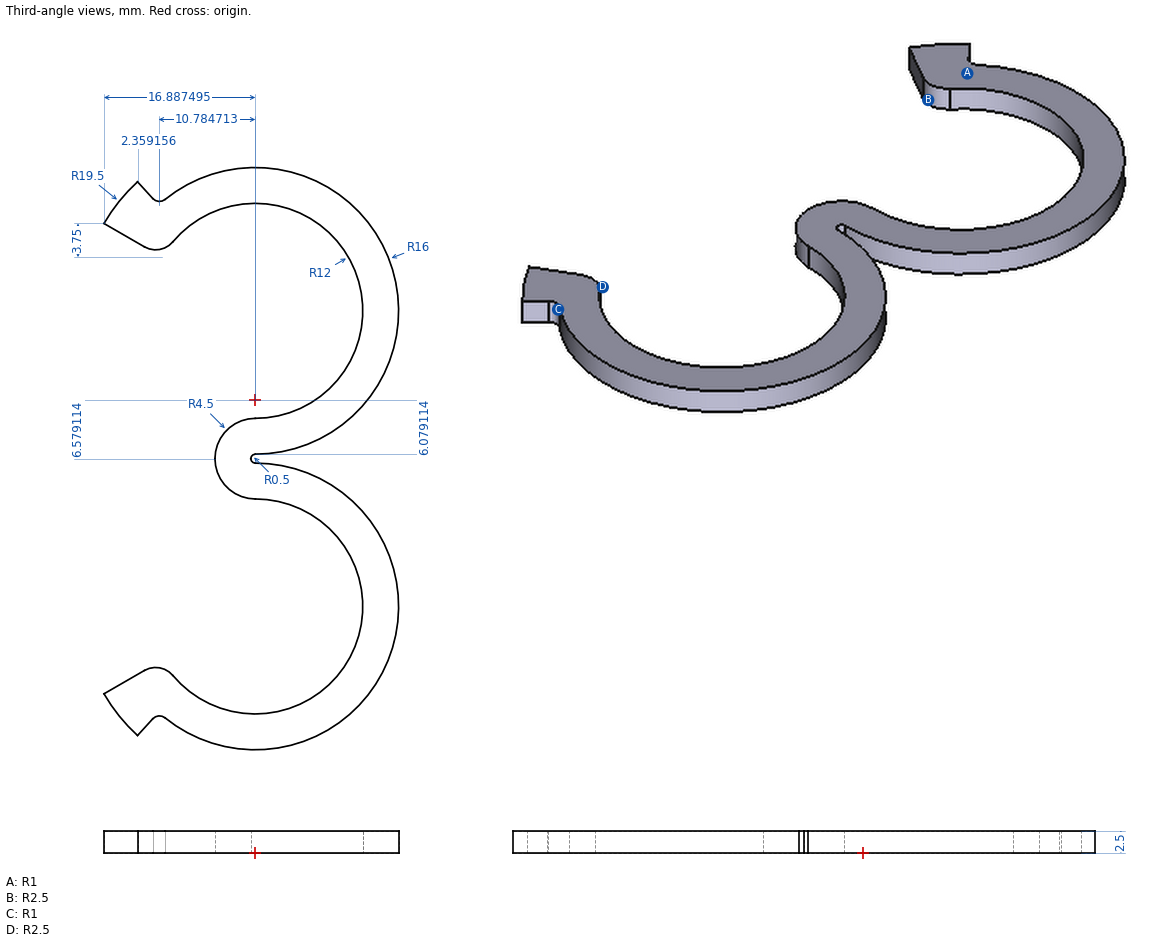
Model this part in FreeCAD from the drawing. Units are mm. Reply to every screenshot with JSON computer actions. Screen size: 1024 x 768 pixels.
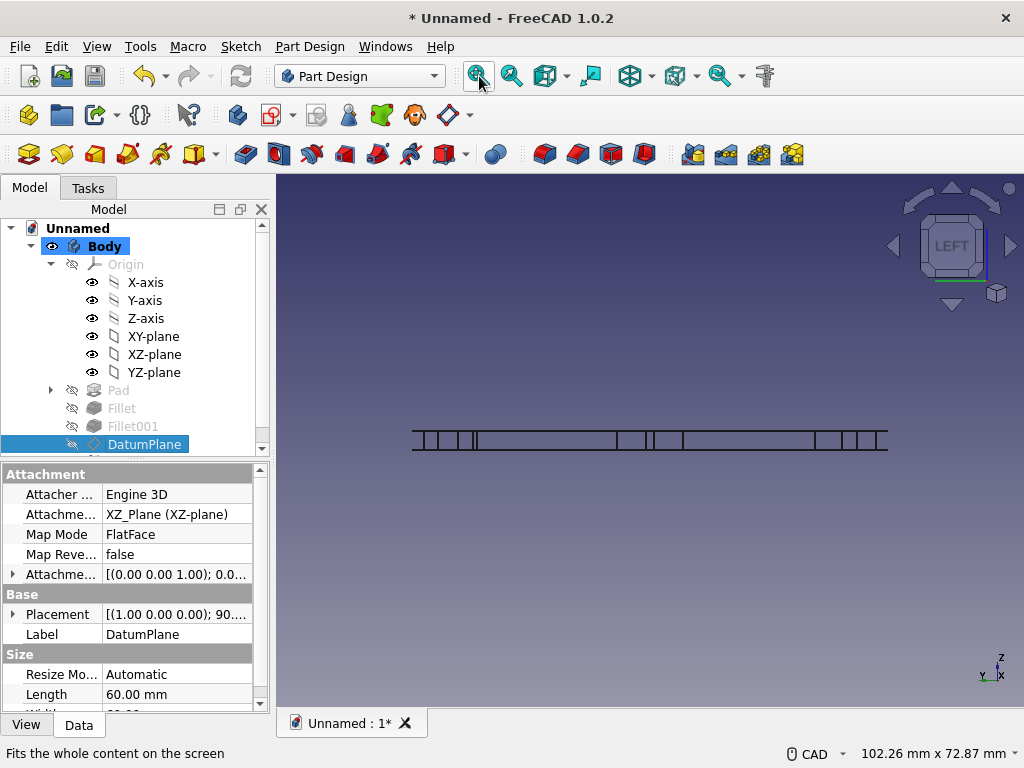
{"action": "key", "text": "0"}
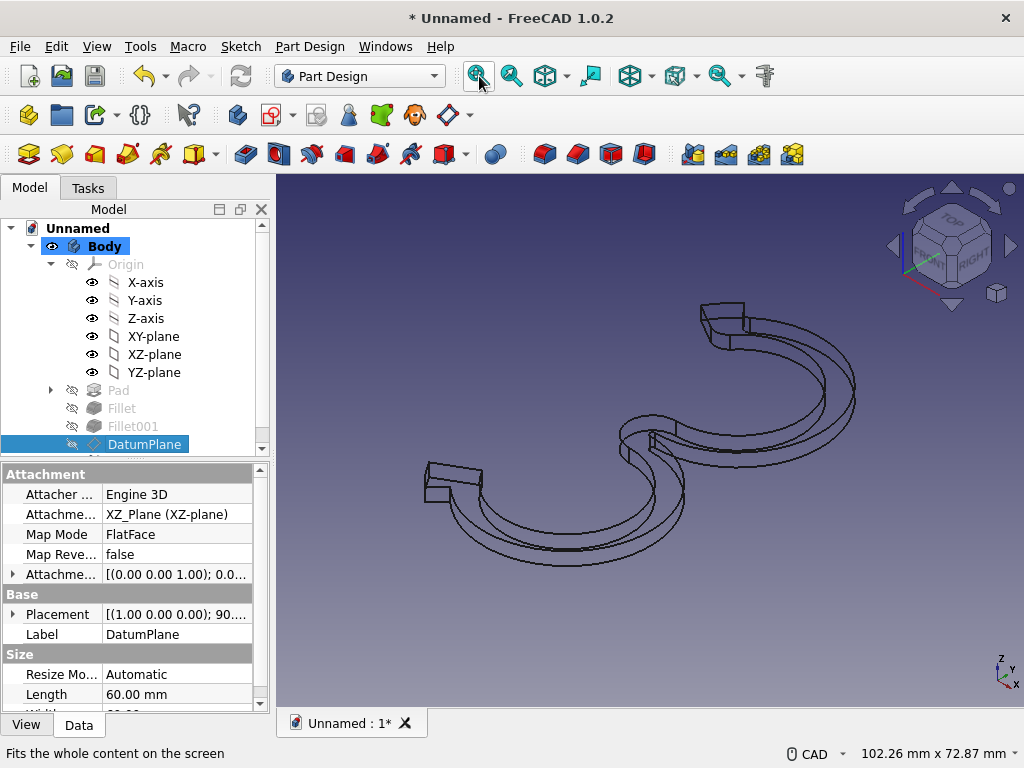
{"action": "scroll", "coordinate": [450, 493], "scroll_direction": "up", "scroll_amount": 4}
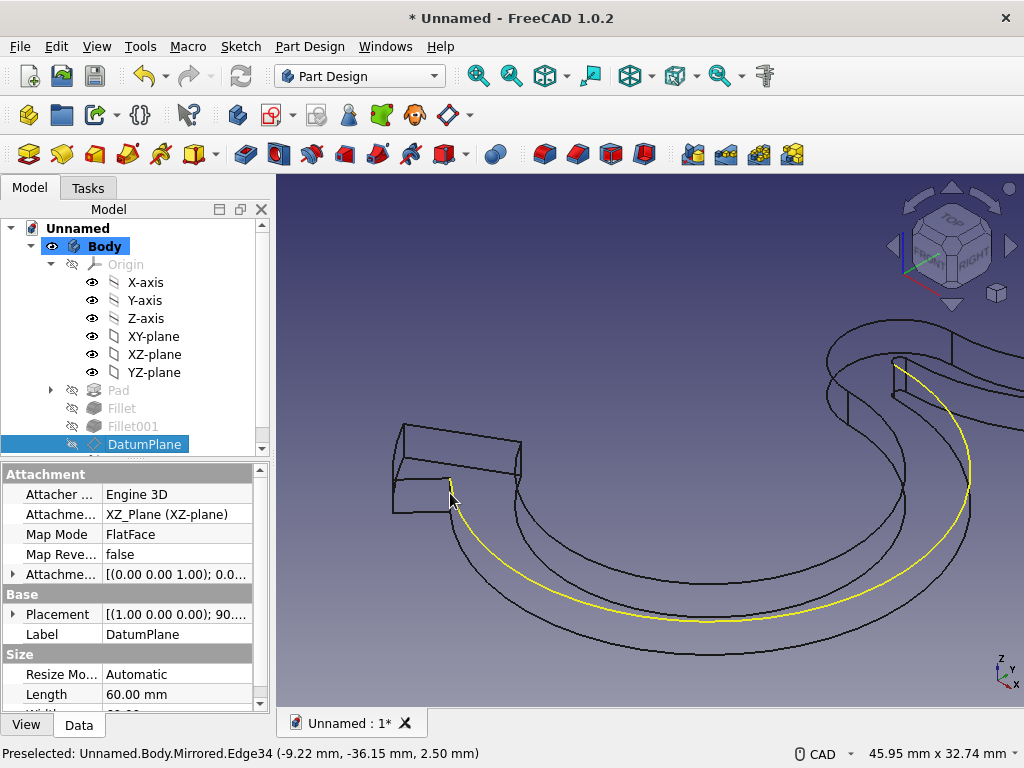
{"action": "left_click", "coordinate": [479, 76]}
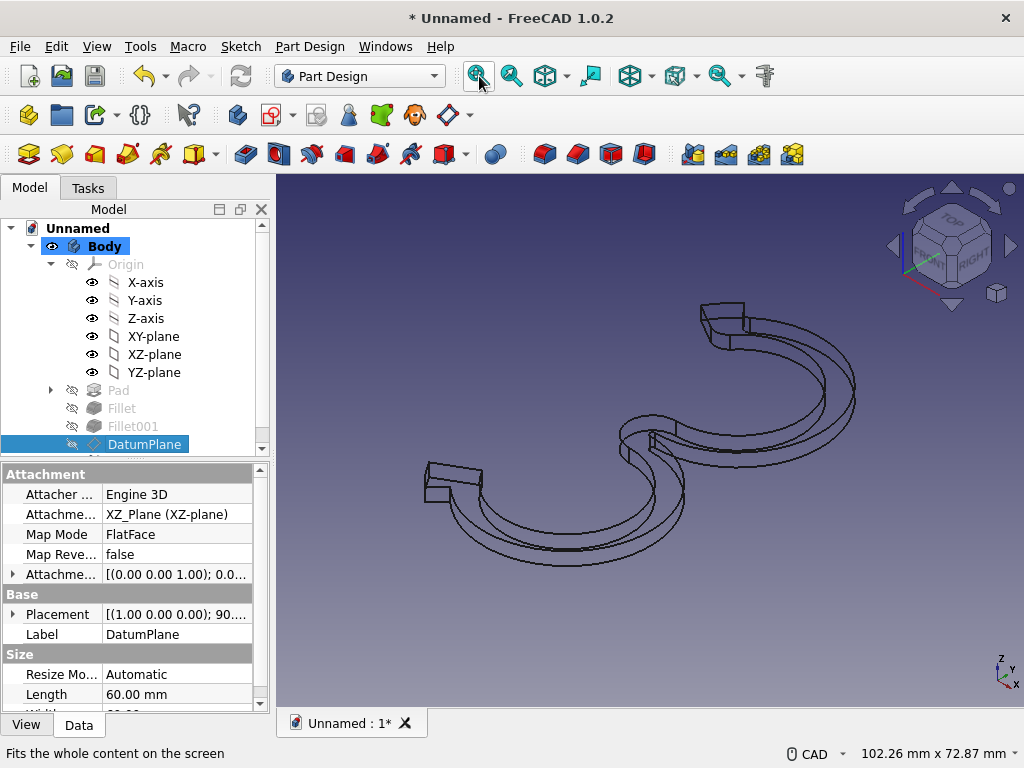
{"action": "key", "text": "2"}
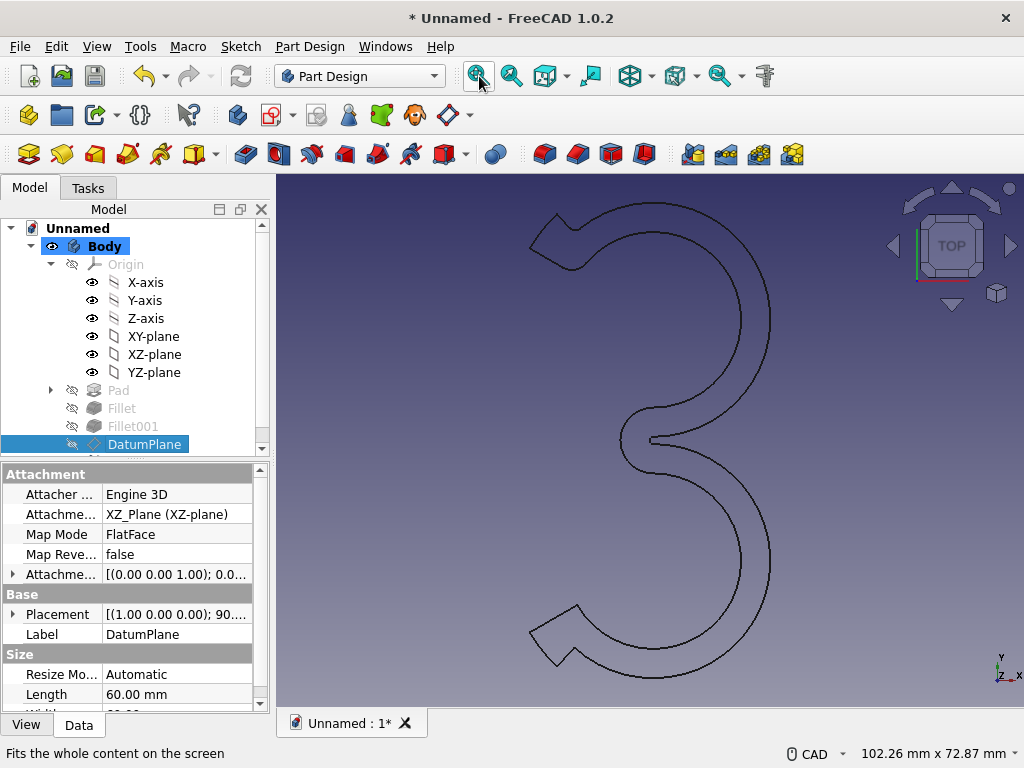
{"action": "scroll", "coordinate": [574, 647], "scroll_direction": "up", "scroll_amount": 4}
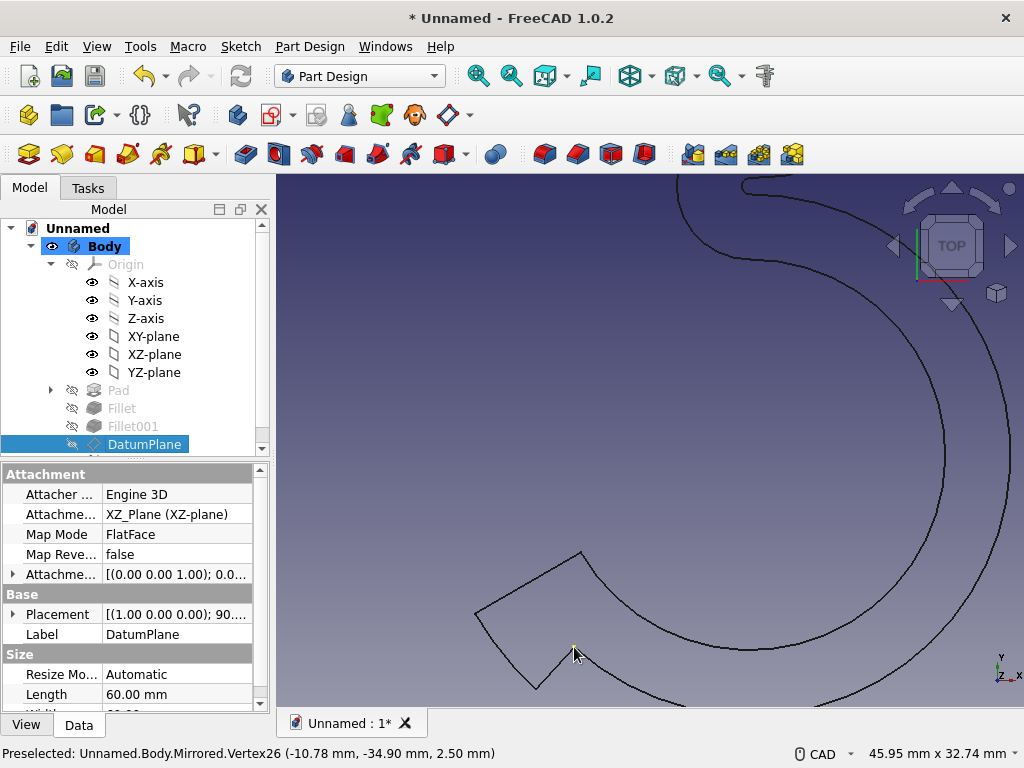
{"action": "left_click", "coordinate": [479, 76]}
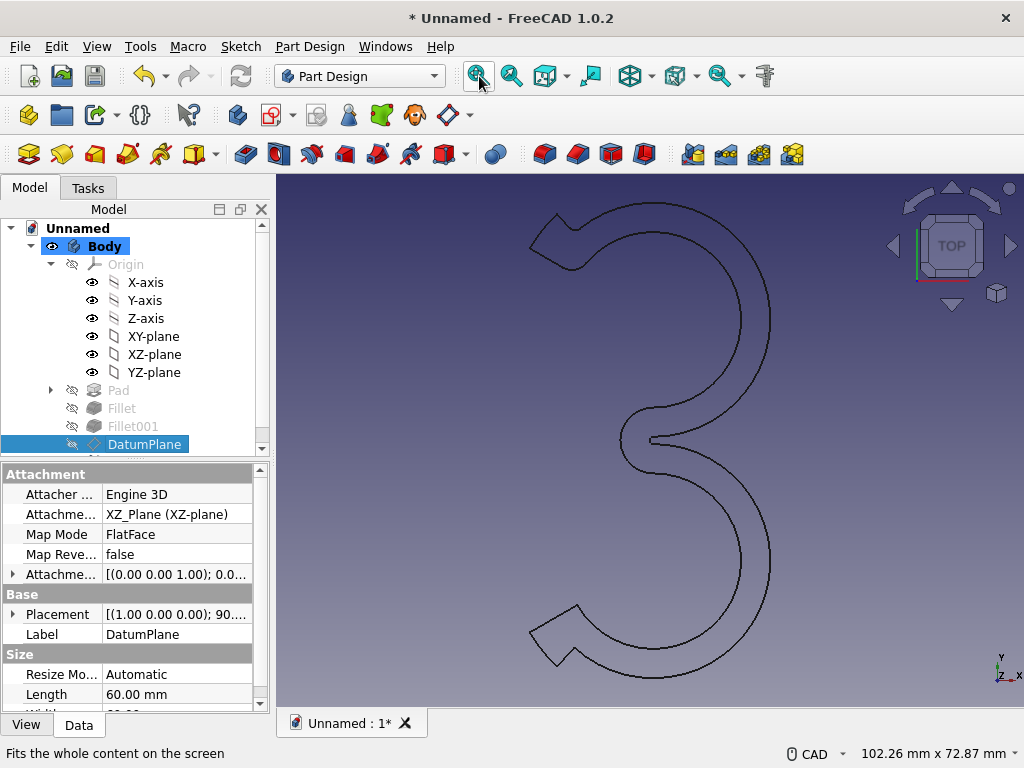
{"action": "key", "text": "1"}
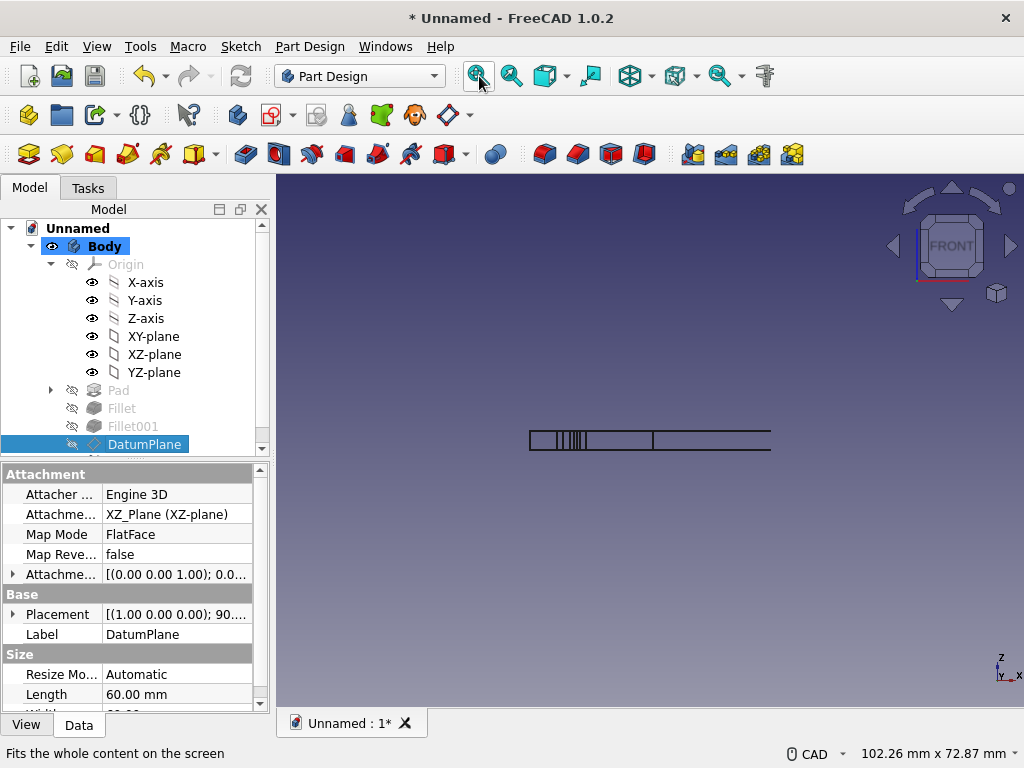
{"action": "left_click", "coordinate": [479, 76]}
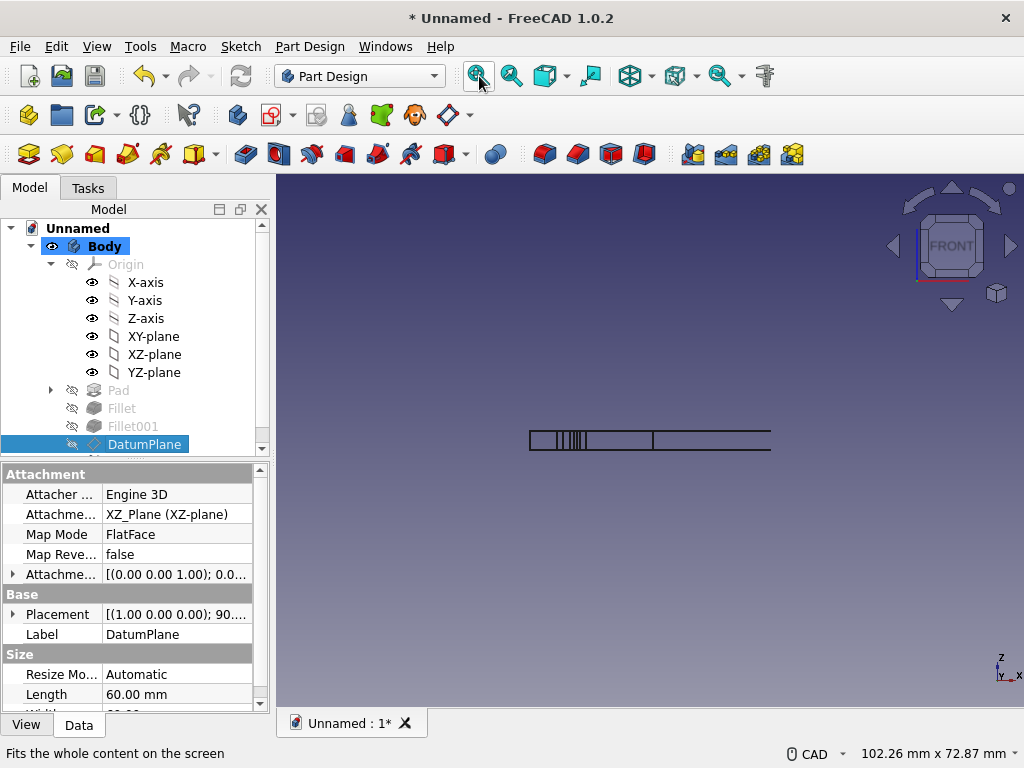
{"action": "left_click", "coordinate": [574, 440]}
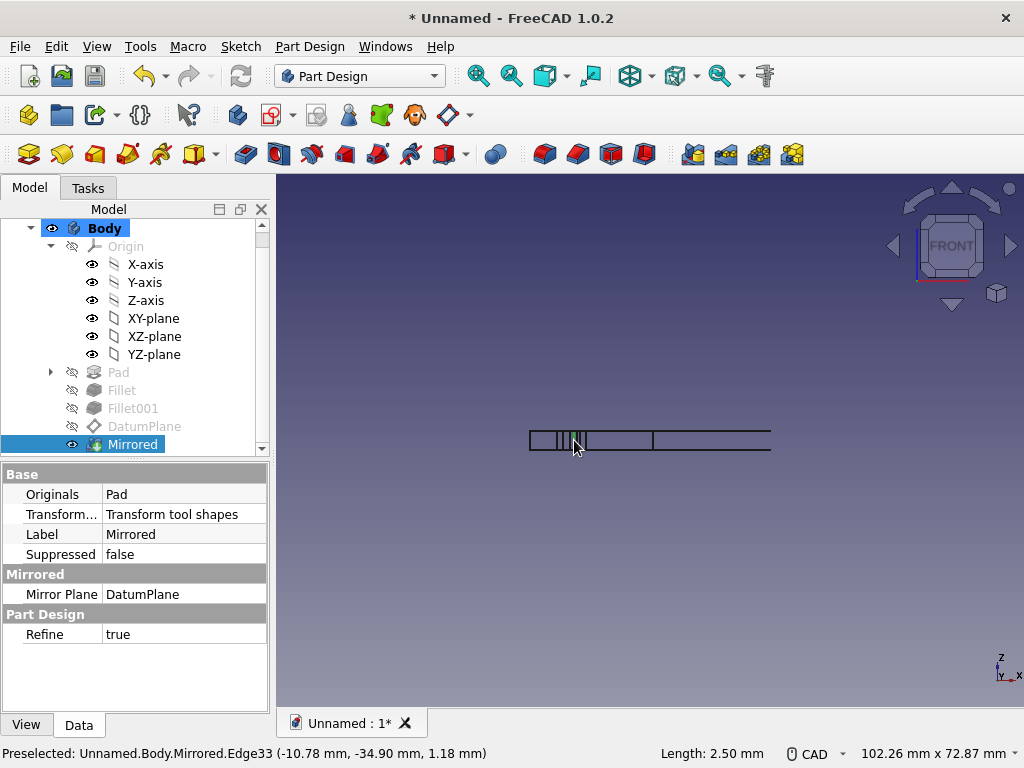
{"action": "key", "text": "v 1"}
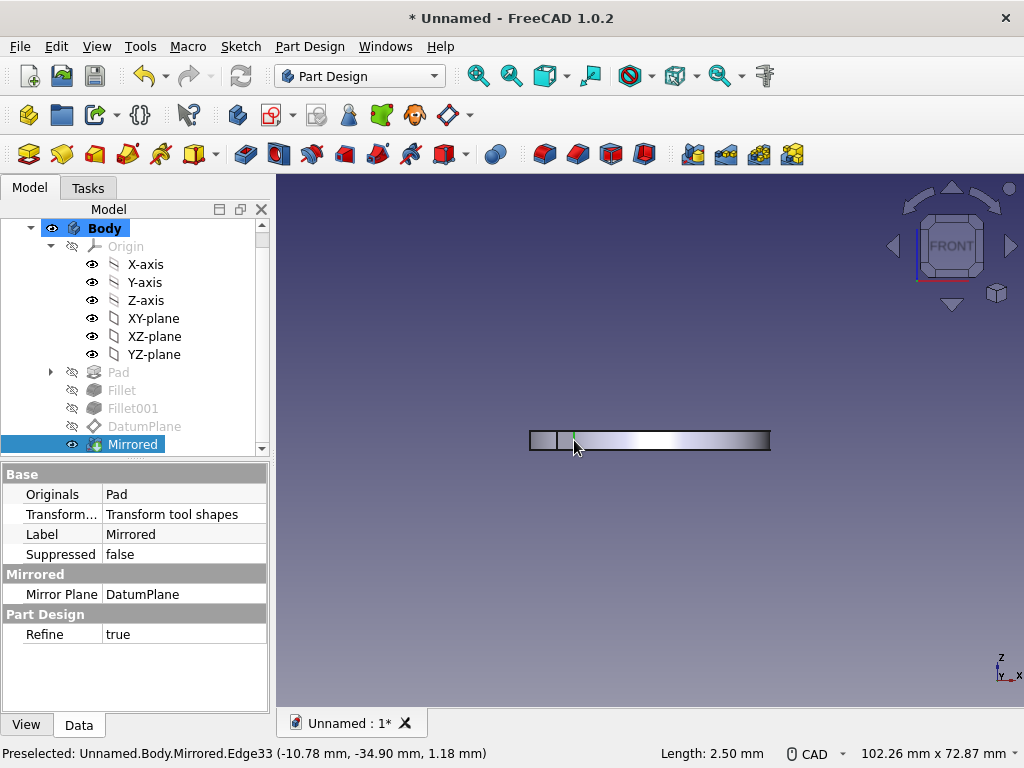
{"action": "left_click", "coordinate": [545, 154]}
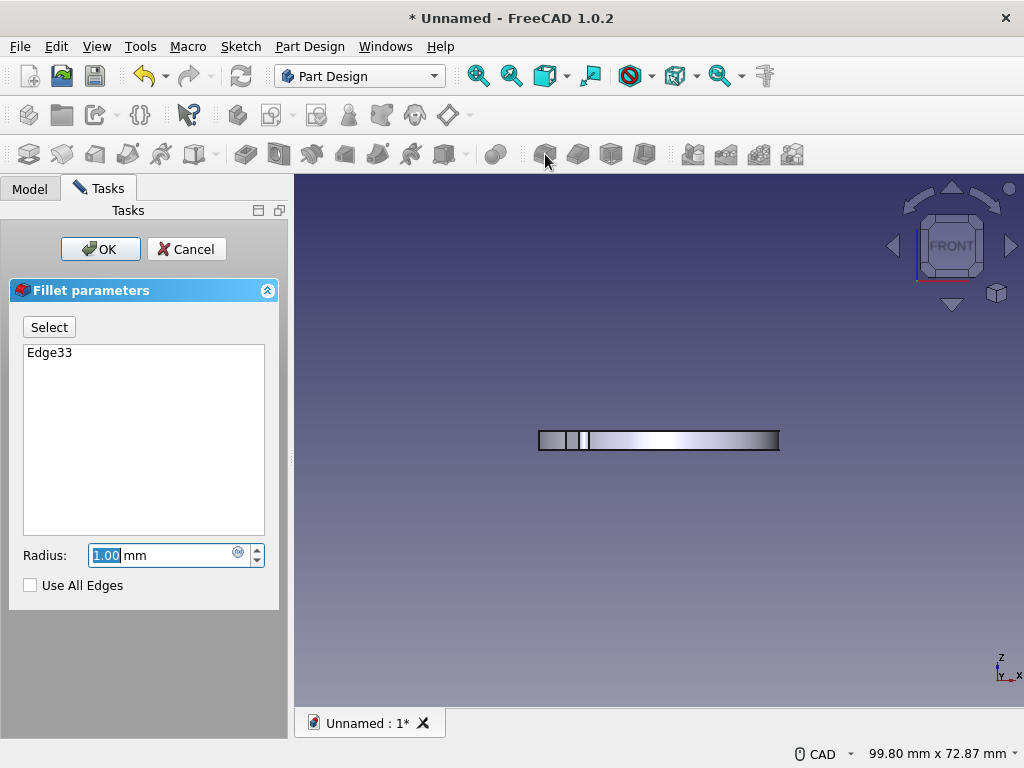
{"action": "type", "text": "1"}
{"action": "key", "text": "Tab"}